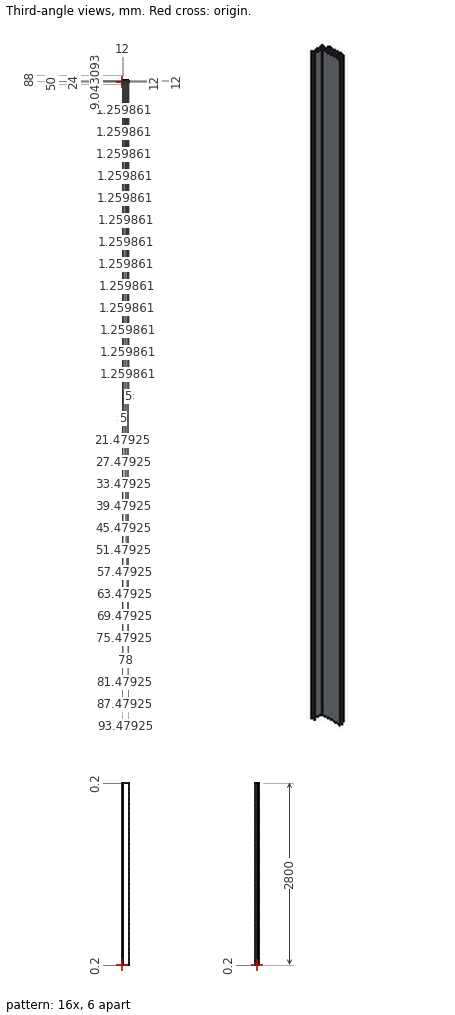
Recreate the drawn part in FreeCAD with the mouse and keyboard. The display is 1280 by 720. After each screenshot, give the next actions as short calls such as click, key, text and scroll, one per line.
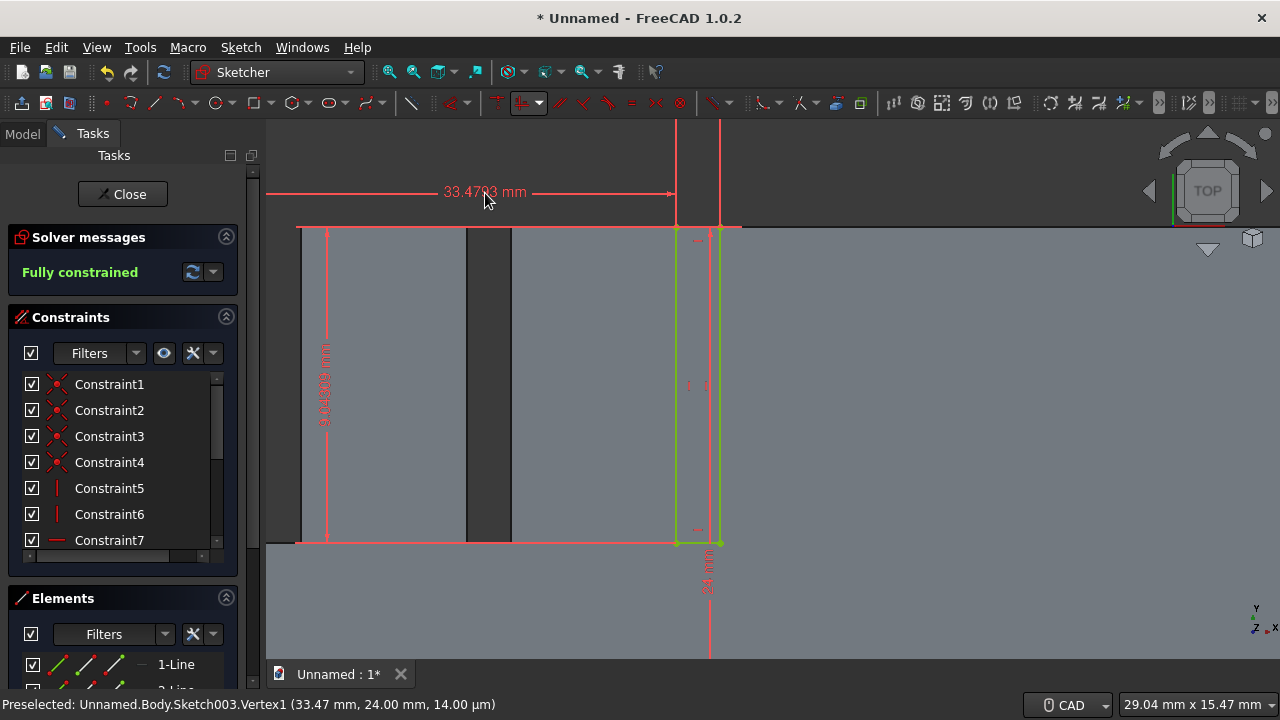
click(123, 194)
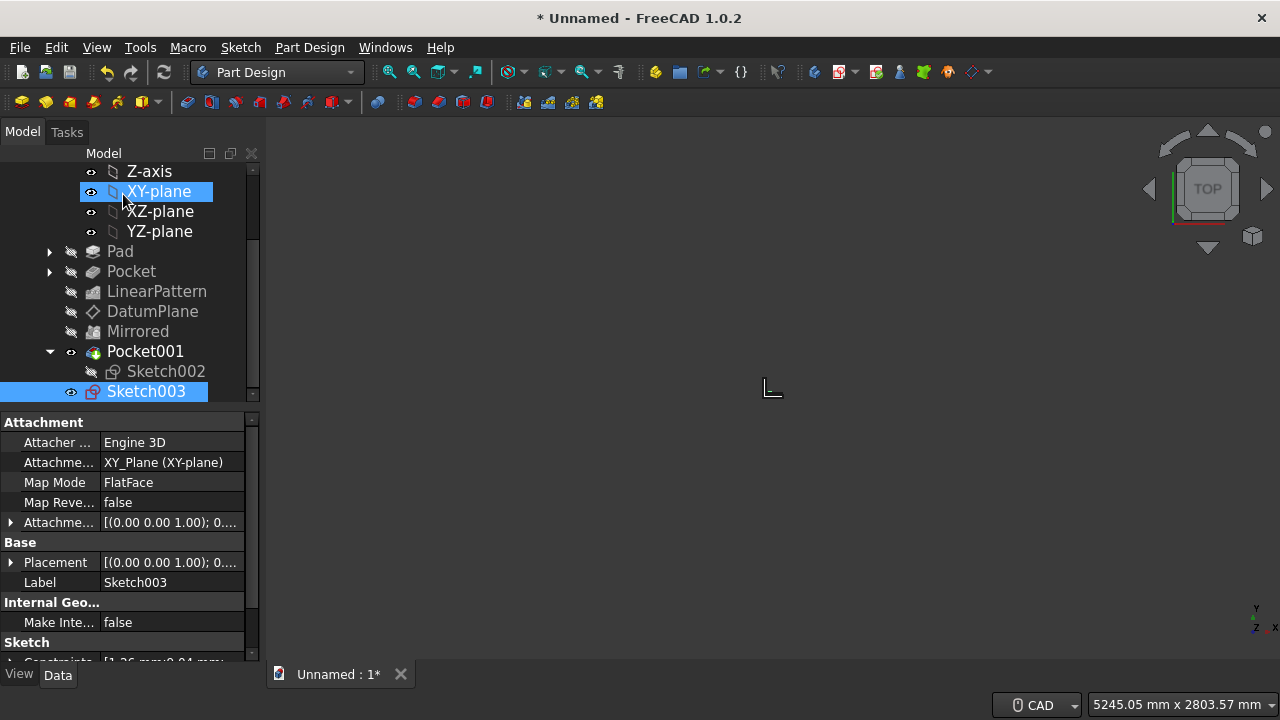
click(188, 102)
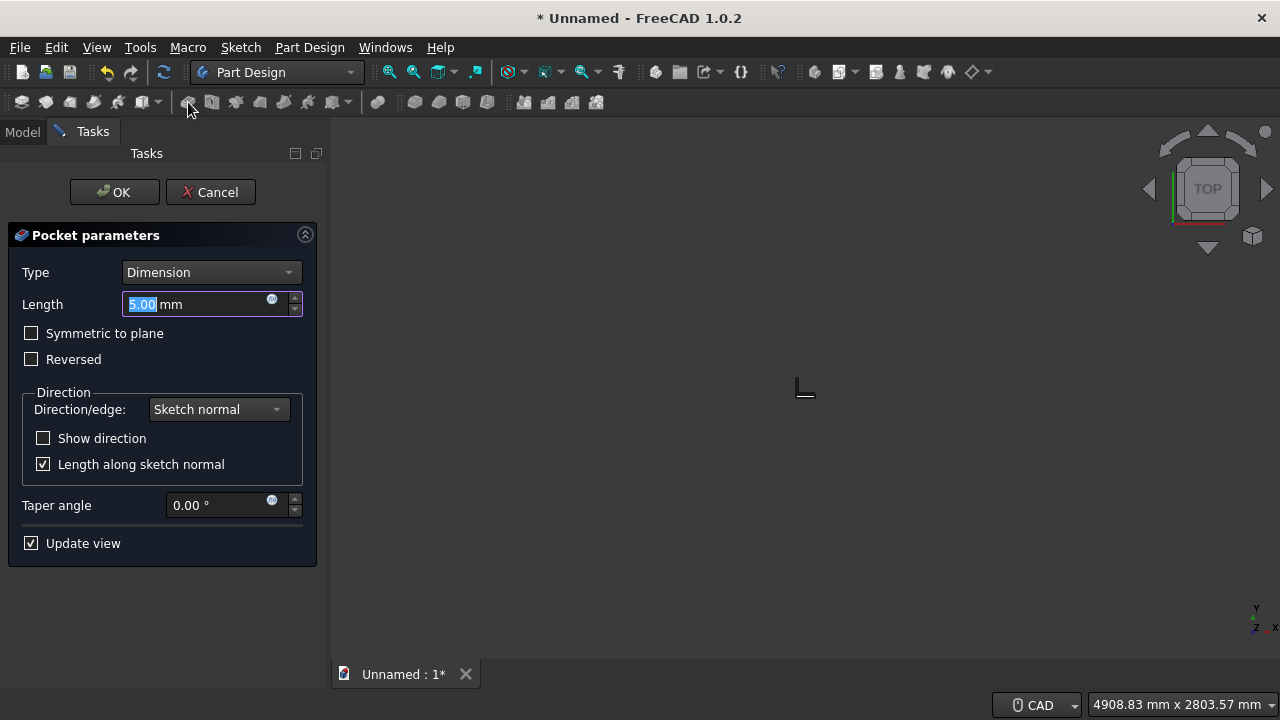
text(0.2)
key(Tab)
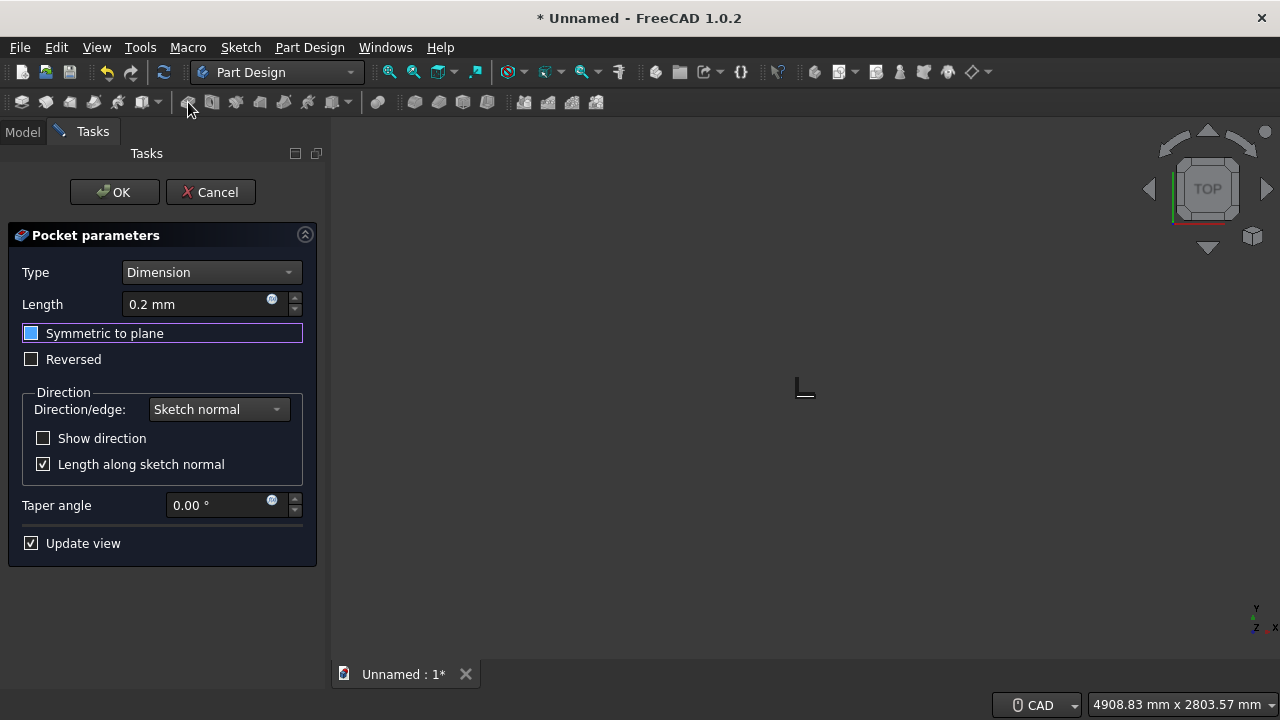
click(30, 359)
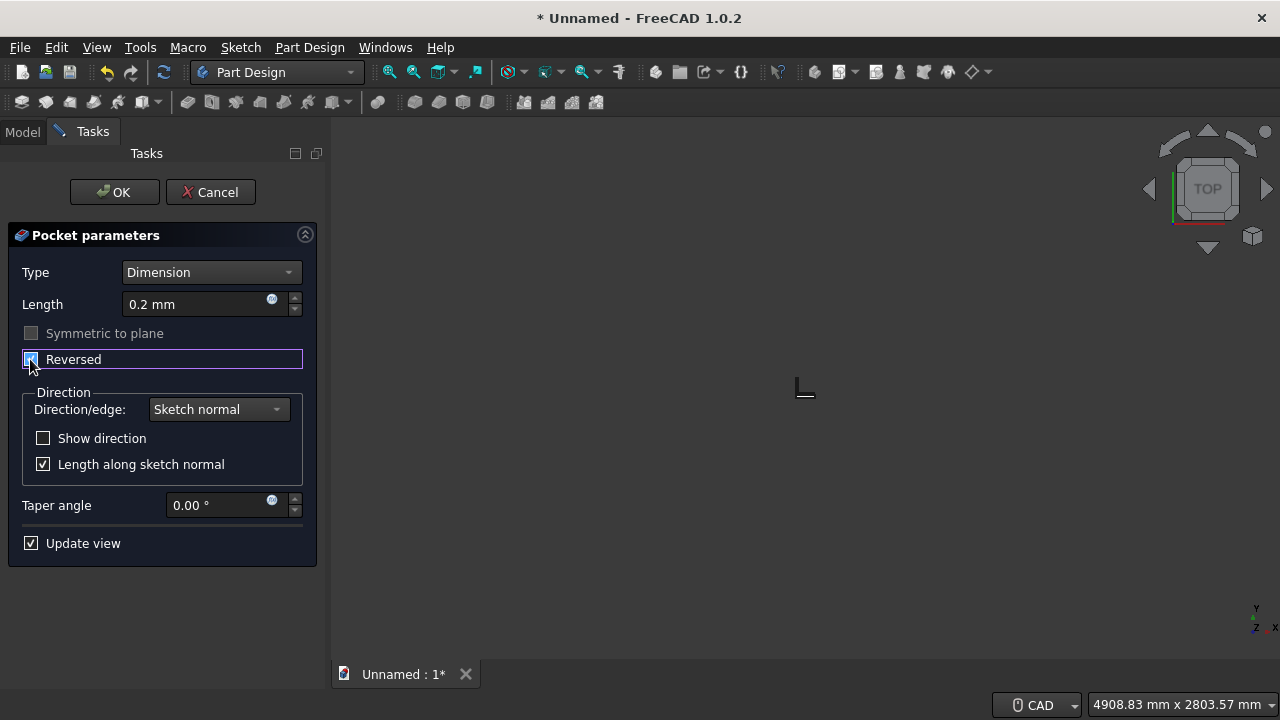
click(115, 192)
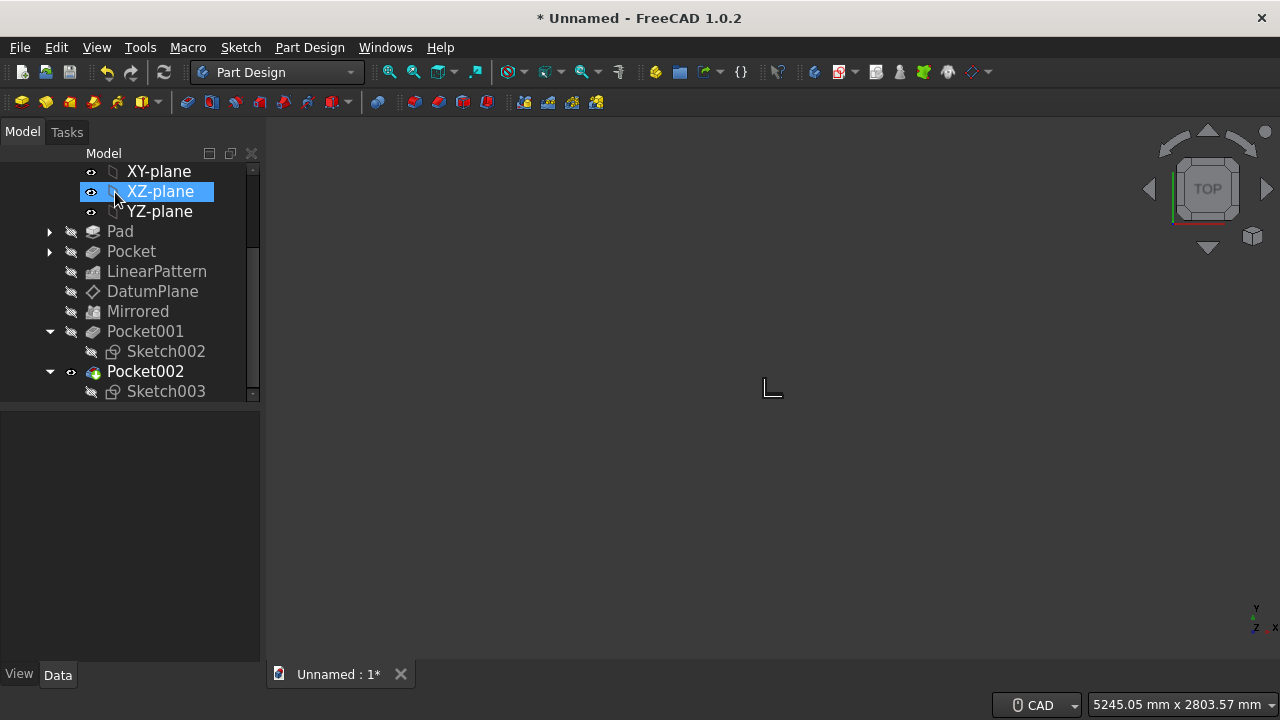
click(390, 72)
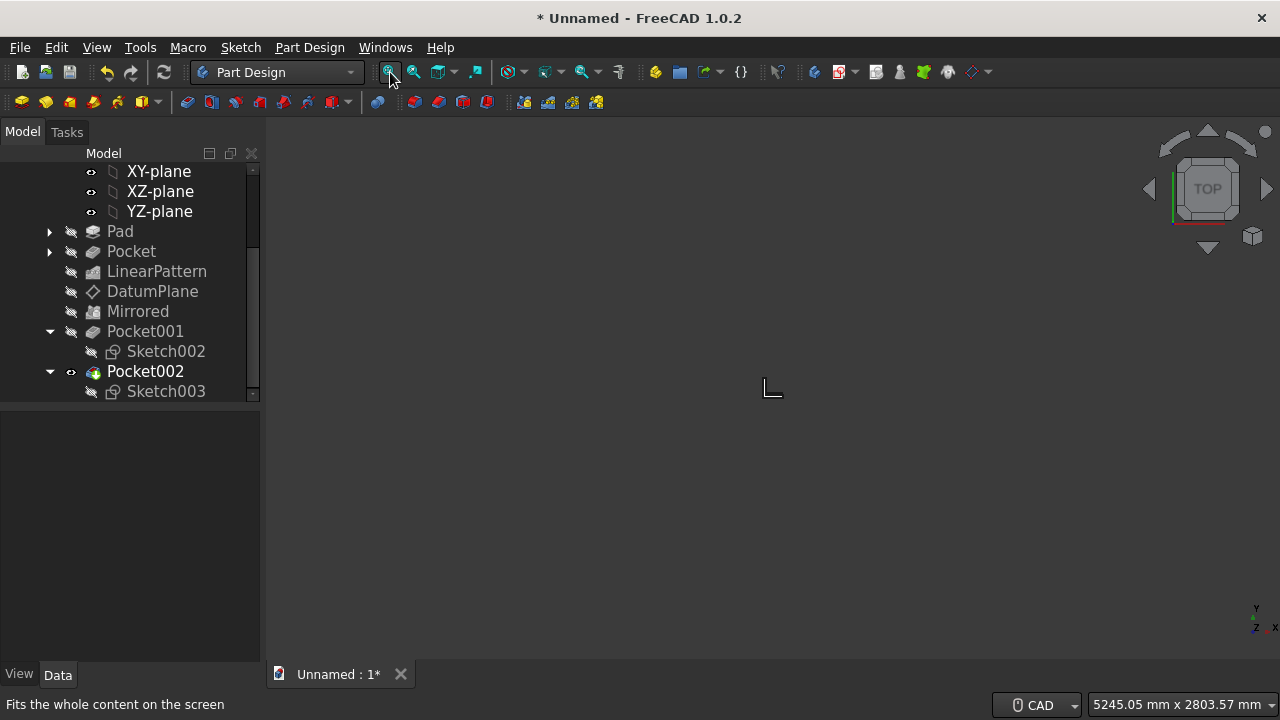
key(5)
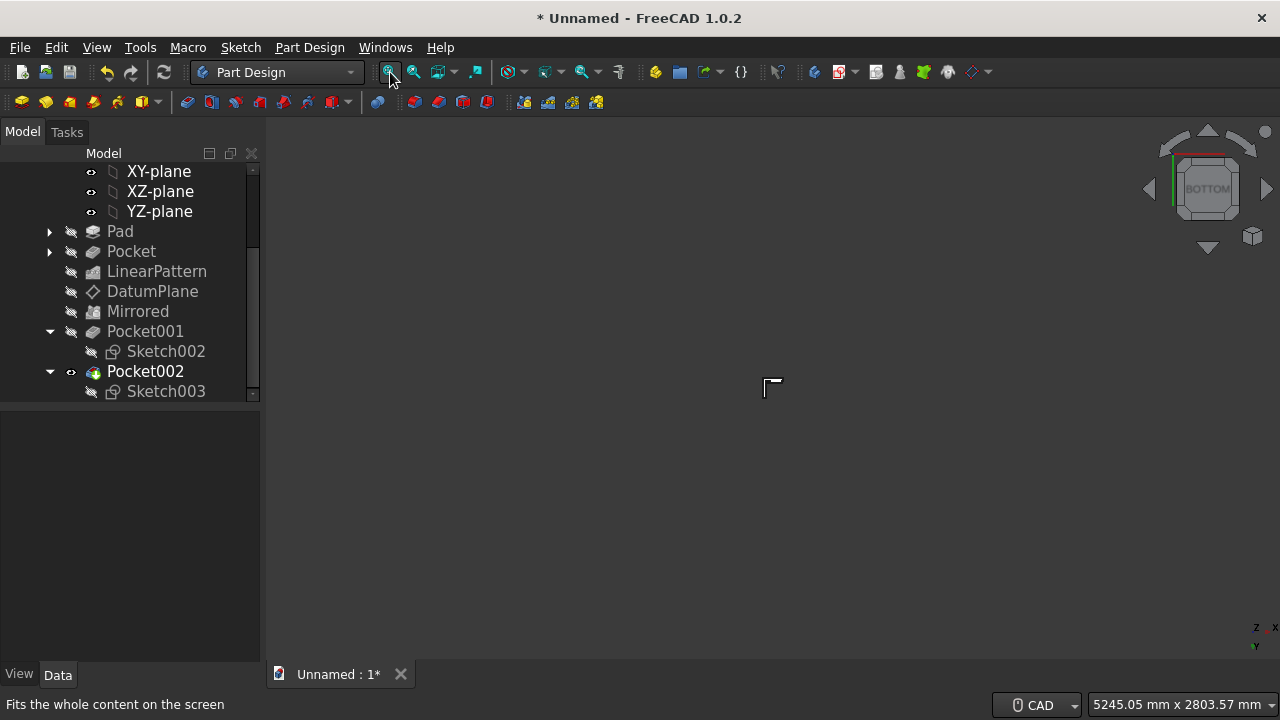
click(390, 72)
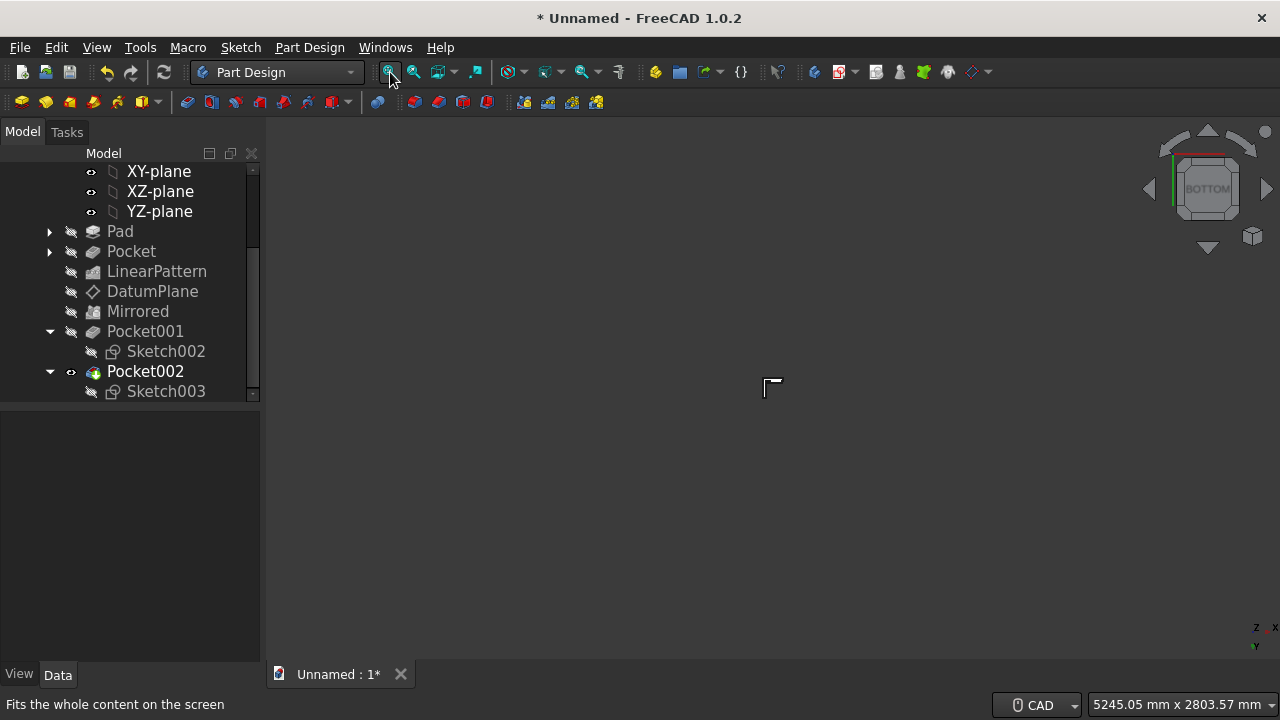
scroll(779, 379, up, 11)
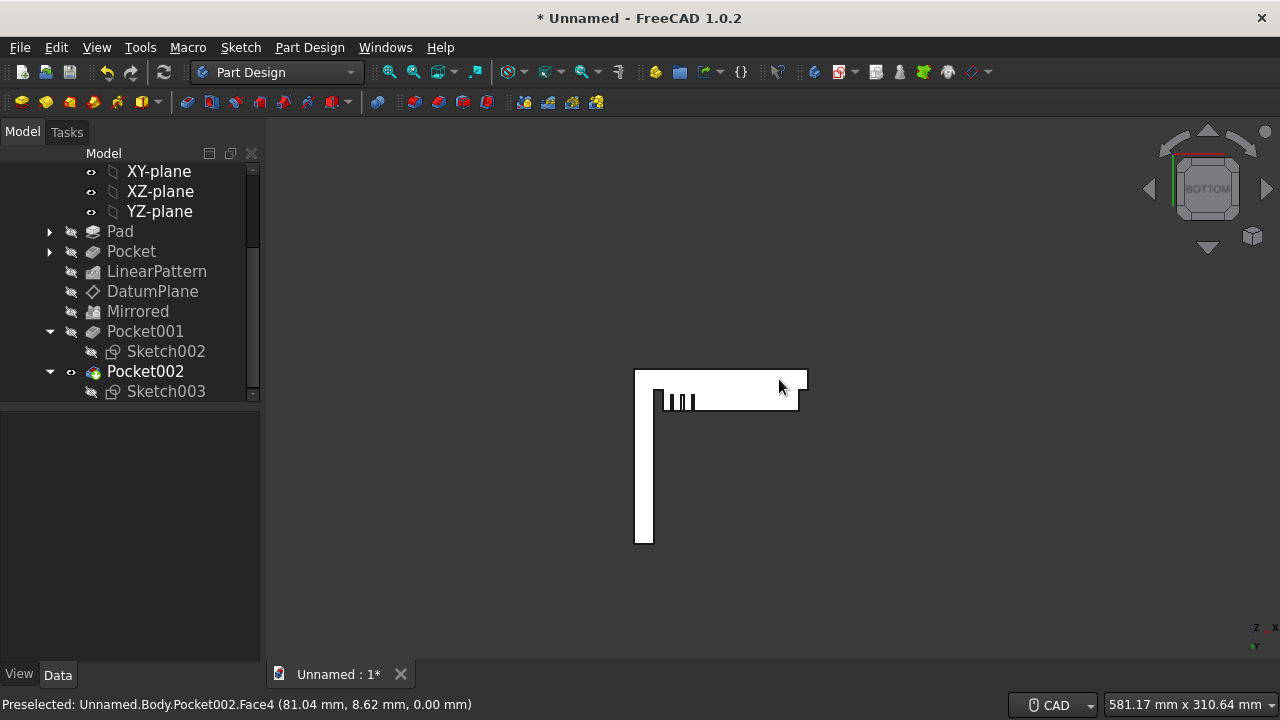
click(771, 381)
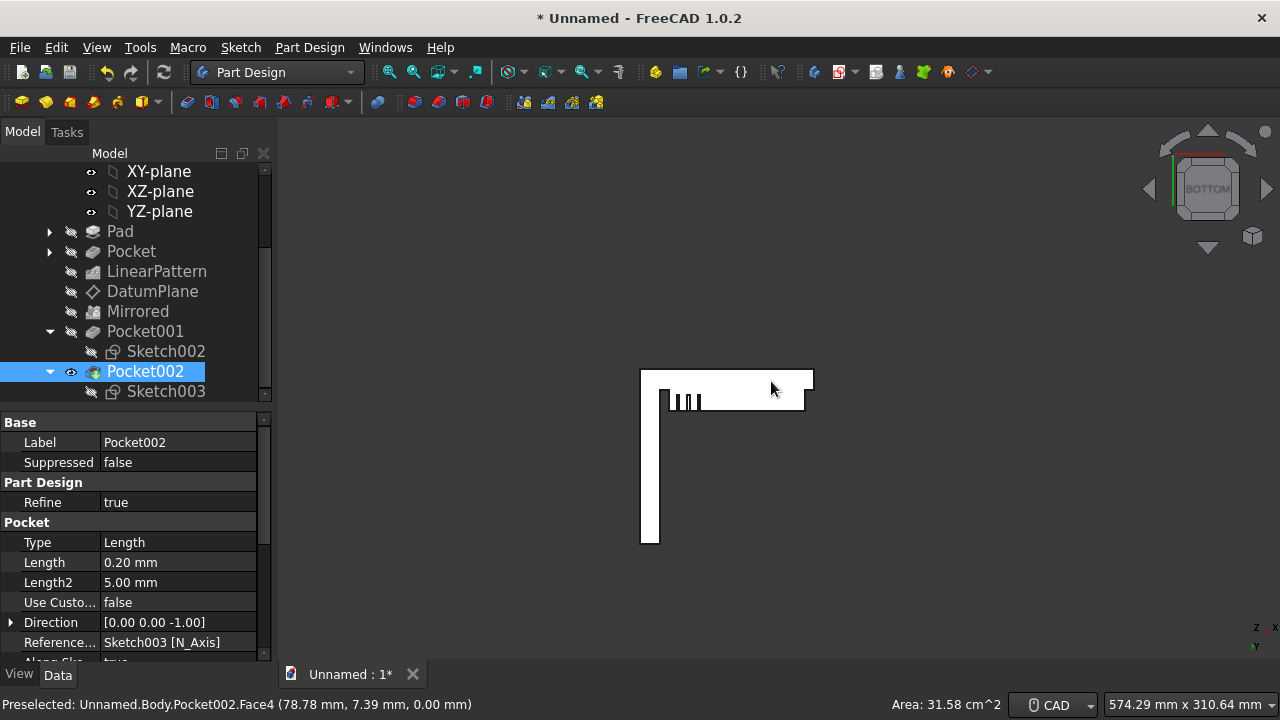
click(840, 72)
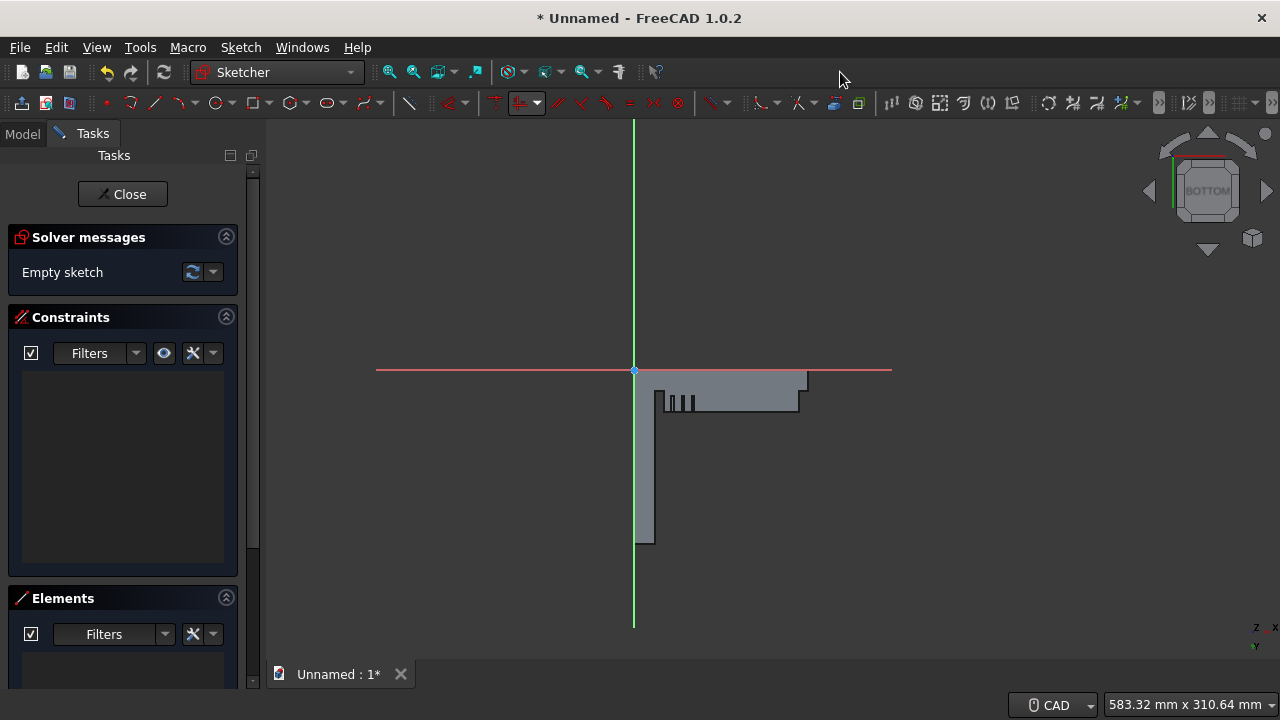
scroll(704, 405, up, 15)